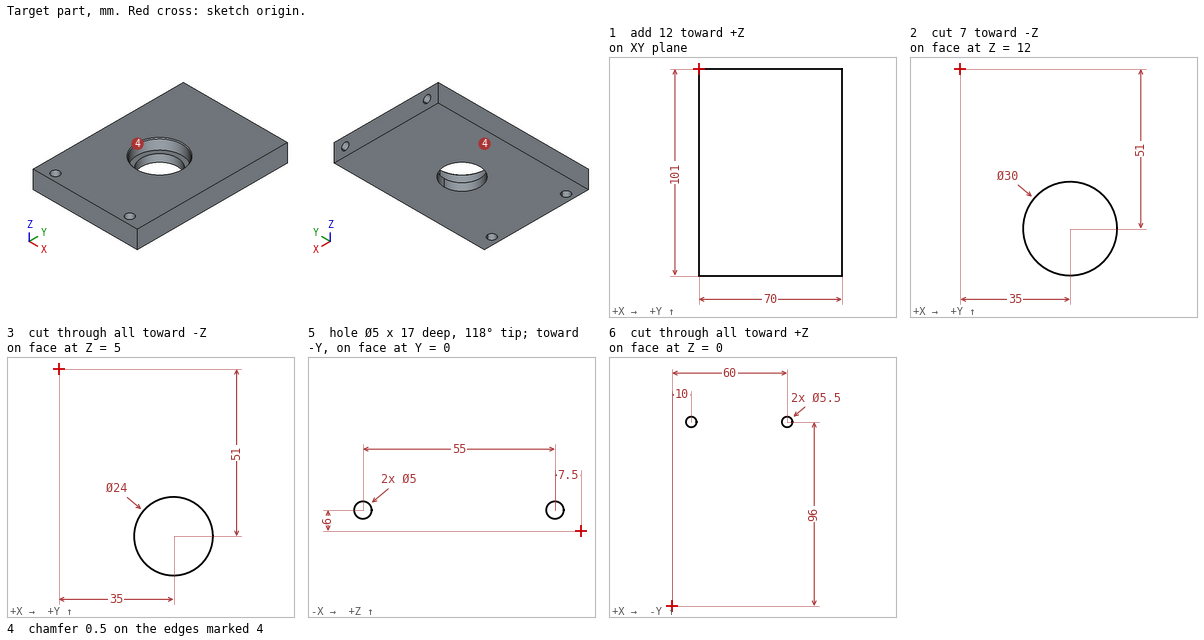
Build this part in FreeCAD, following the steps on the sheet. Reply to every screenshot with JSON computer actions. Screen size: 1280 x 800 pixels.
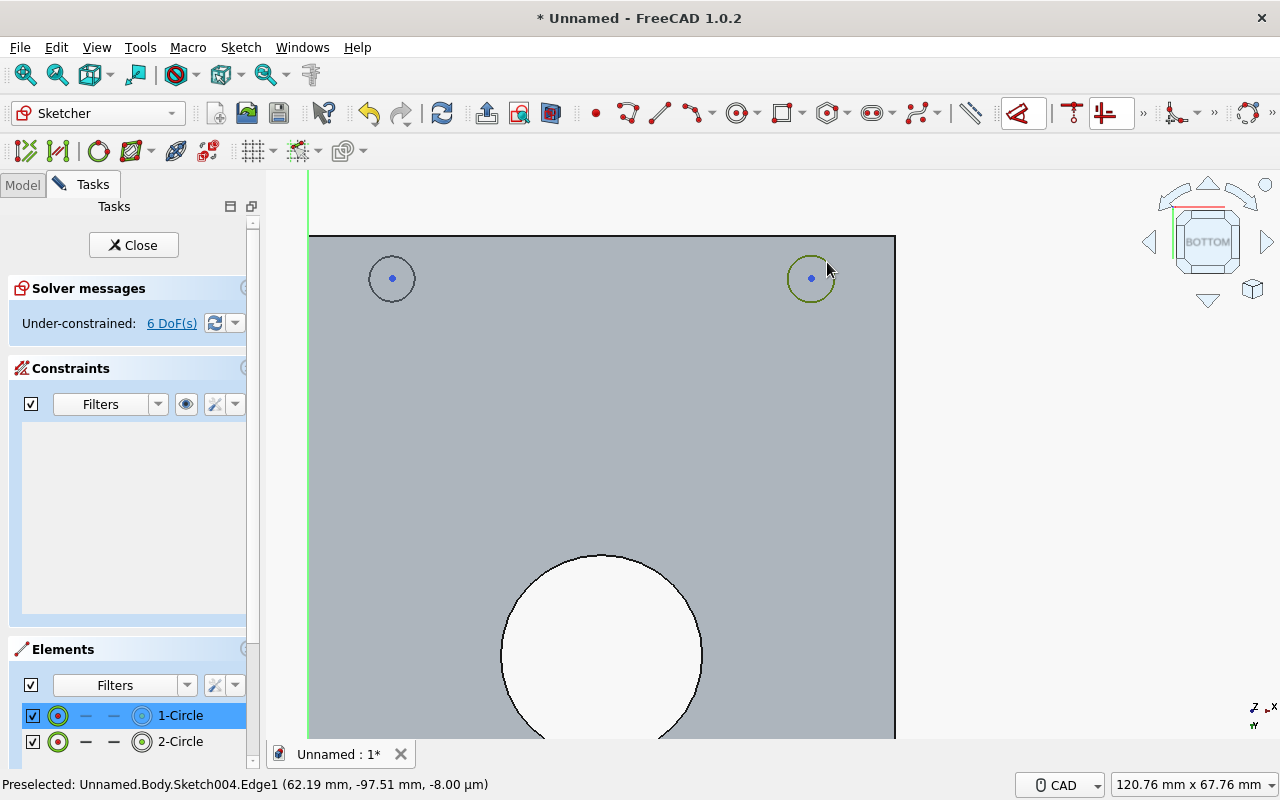
{"action": "left_click", "coordinate": [408, 263]}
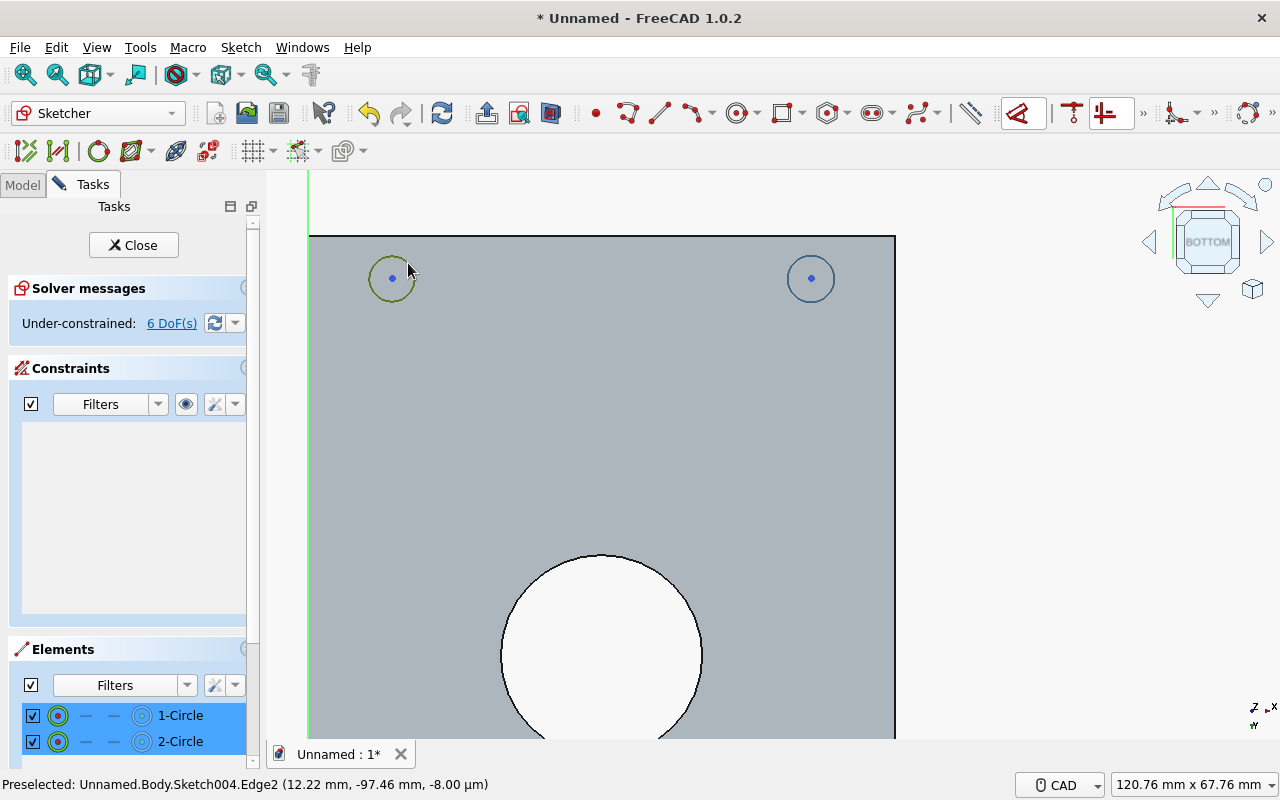
{"action": "key", "text": "e"}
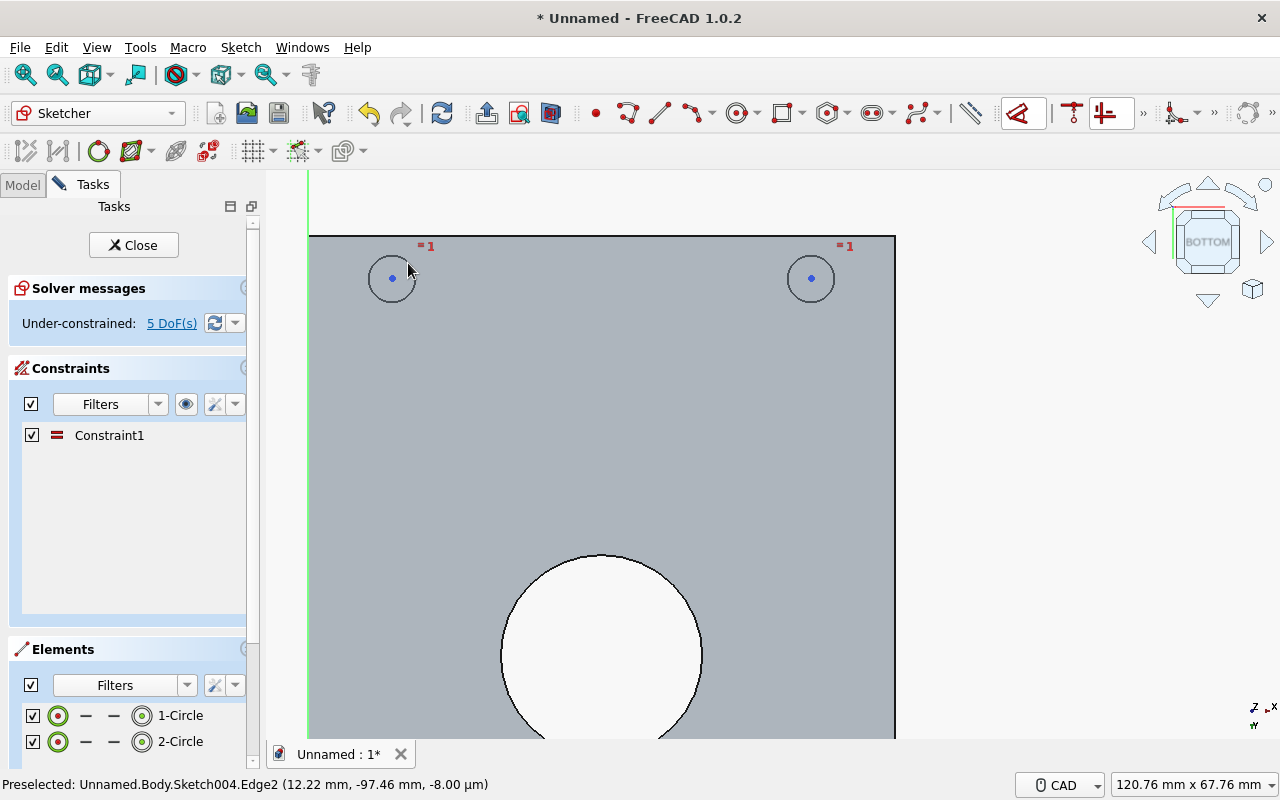
{"action": "left_click", "coordinate": [811, 279]}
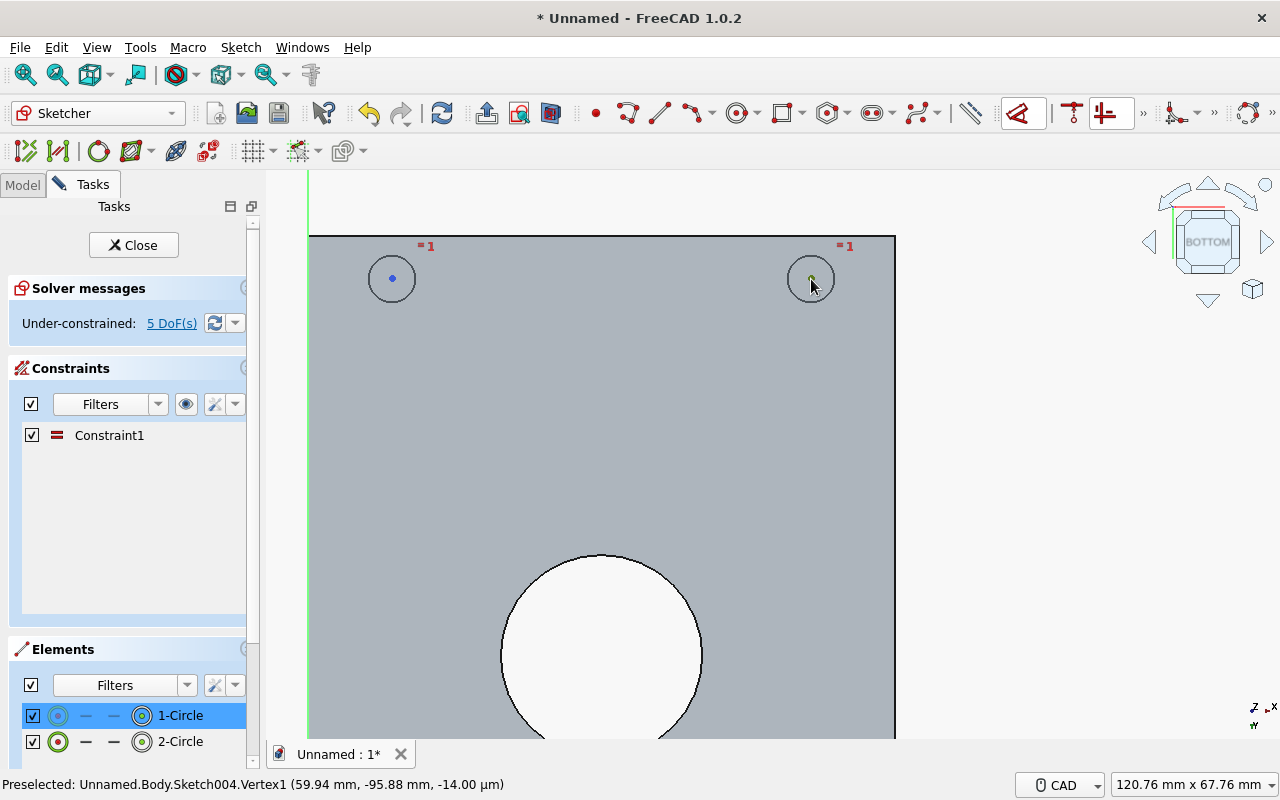
{"action": "left_click", "coordinate": [392, 279]}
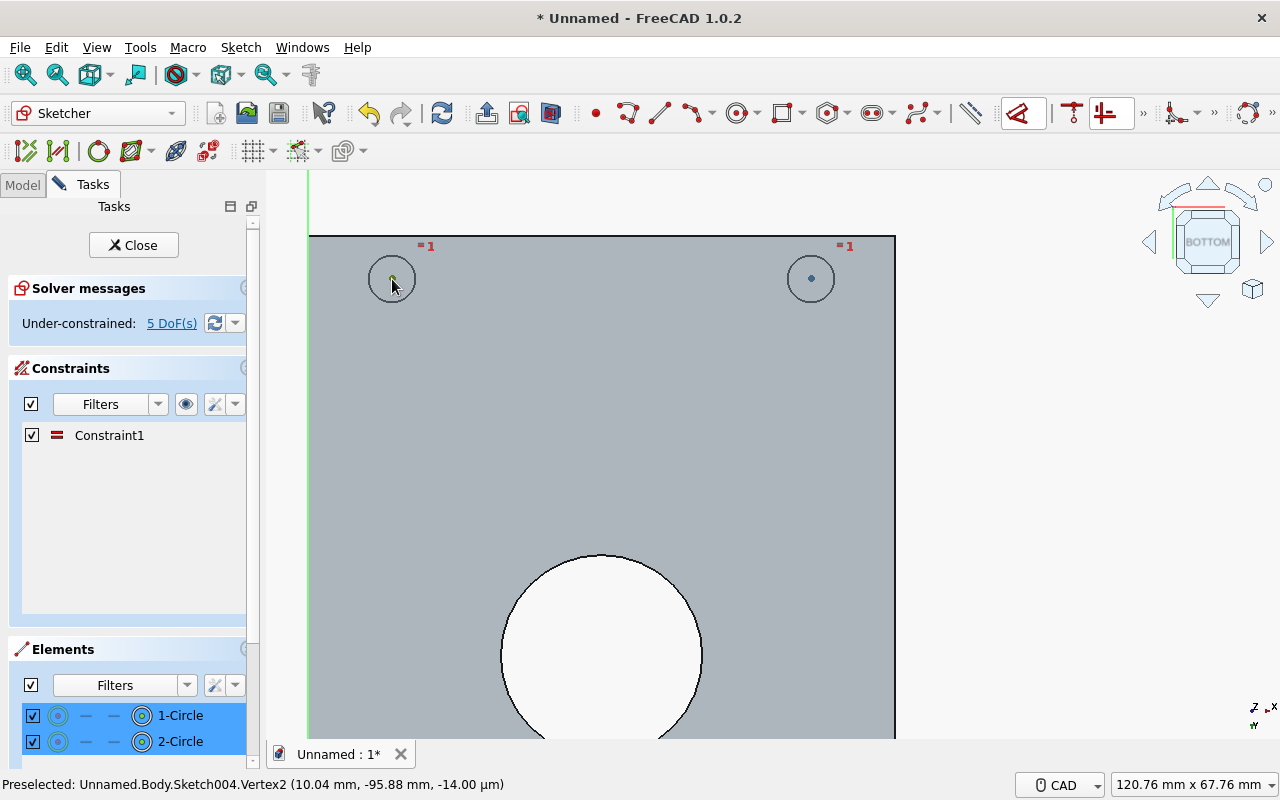
{"action": "key", "text": "h"}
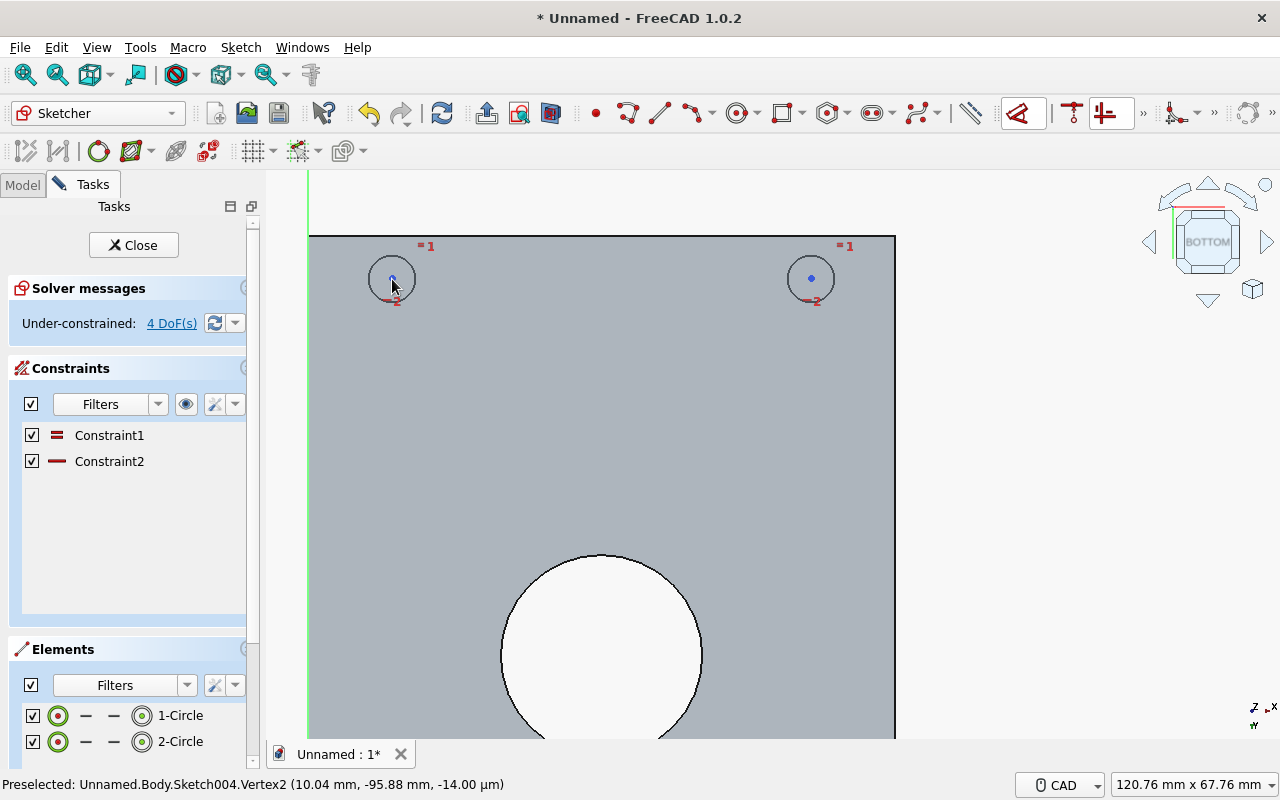
{"action": "left_click", "coordinate": [827, 262]}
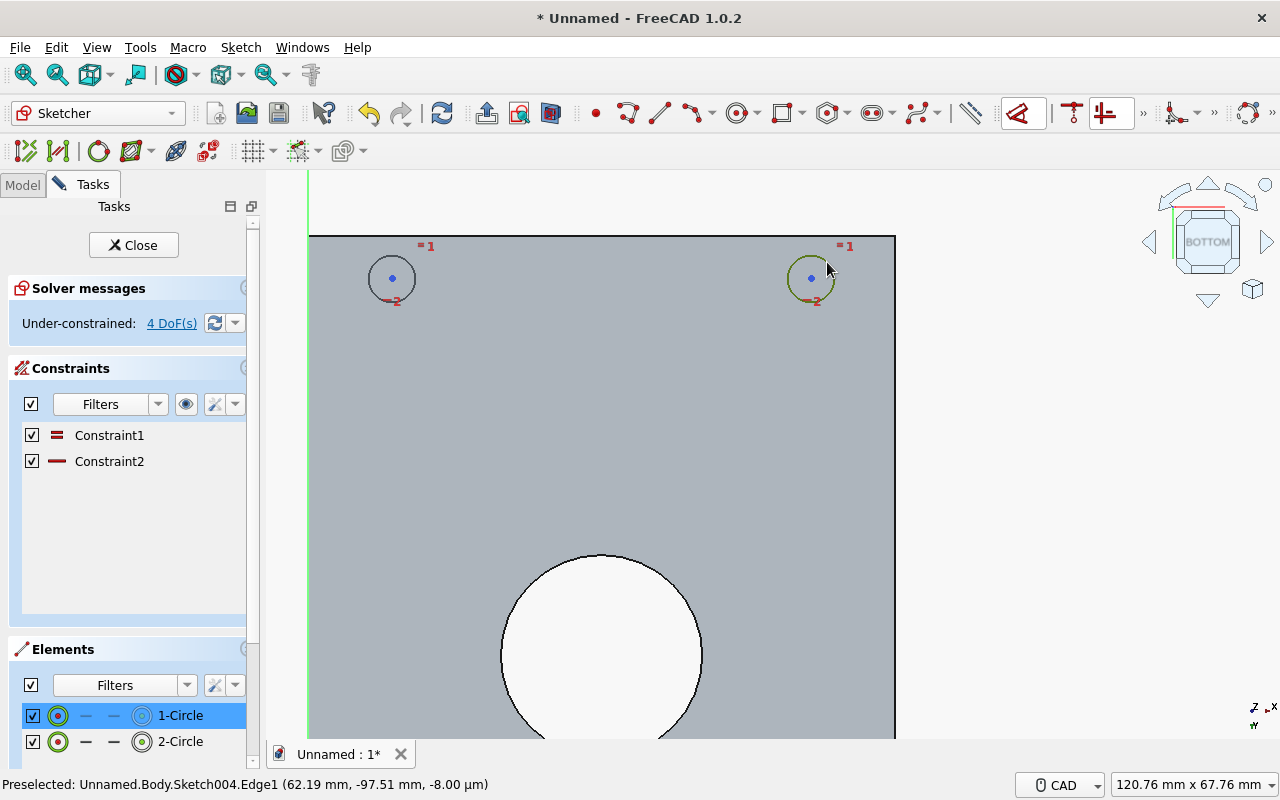
{"action": "key", "text": "k o"}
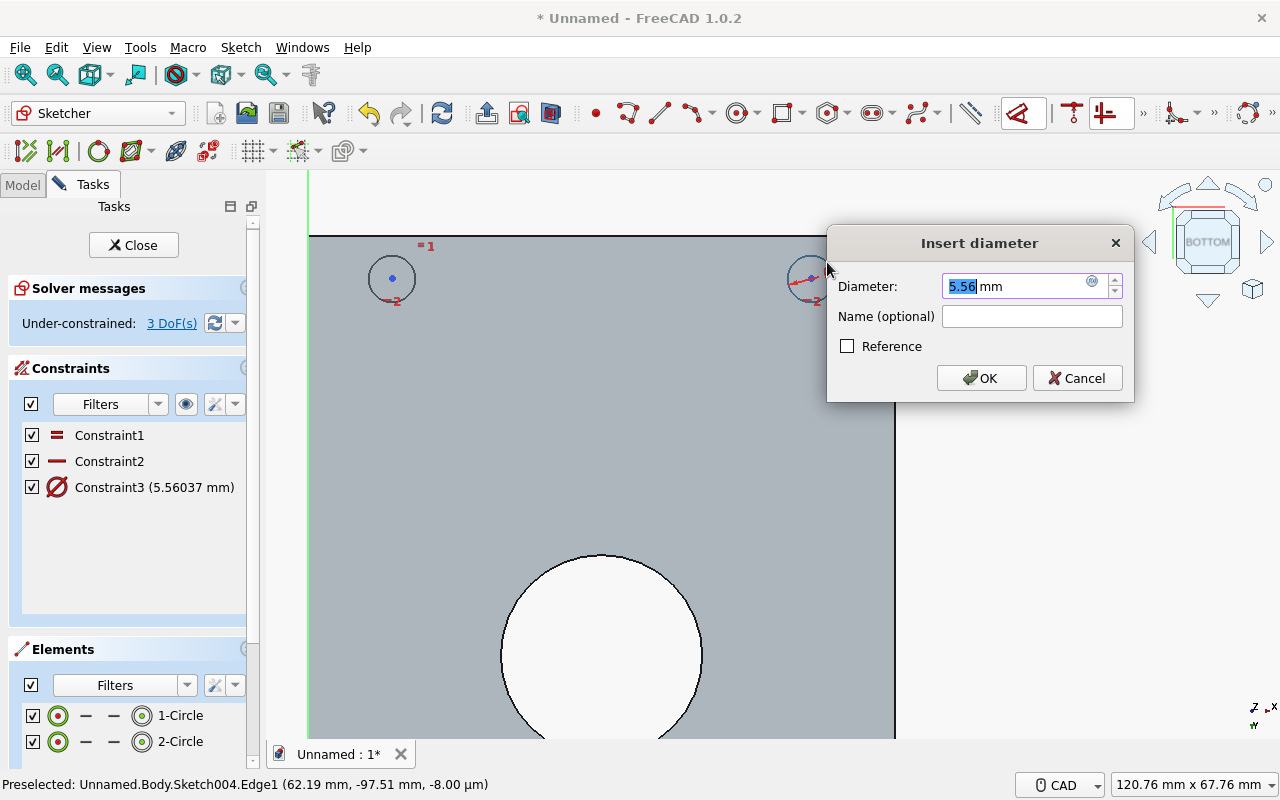
{"action": "type", "text": "5.5"}
{"action": "key", "text": "Return"}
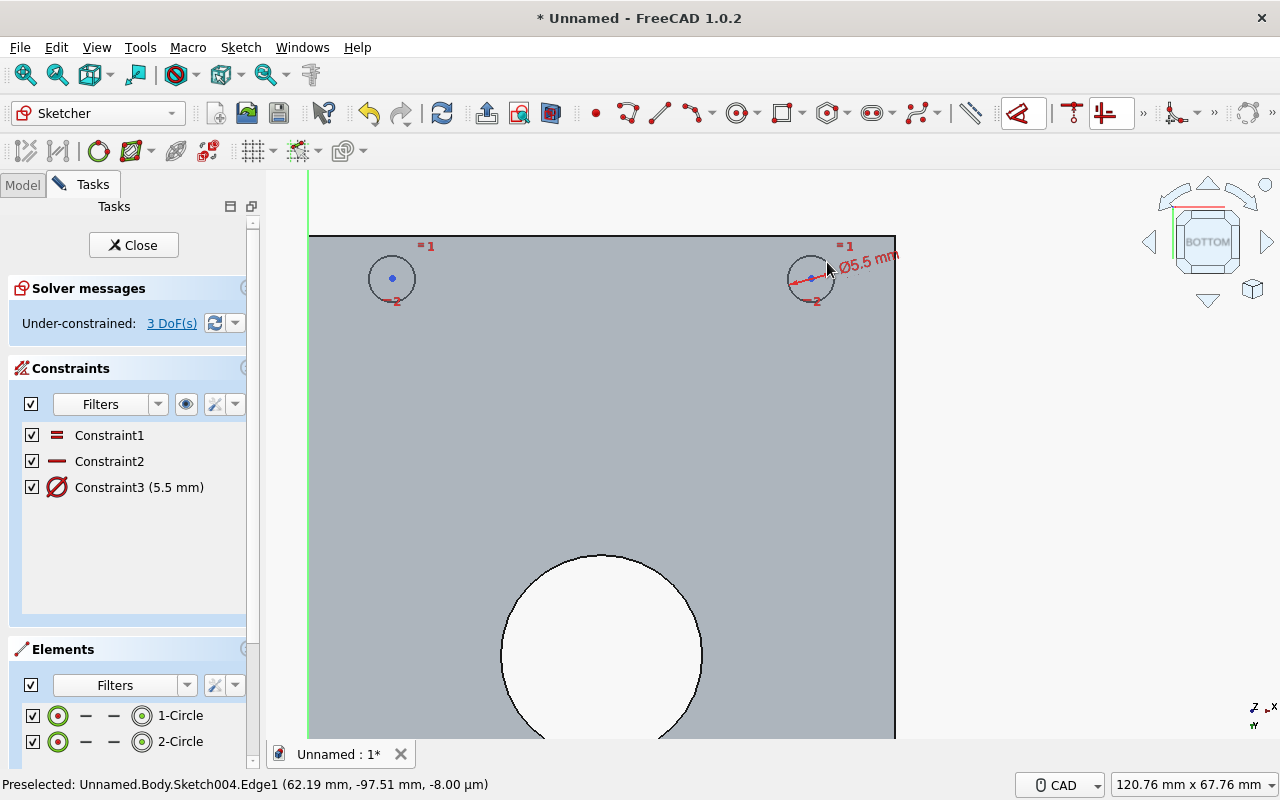
{"action": "left_click", "coordinate": [811, 279]}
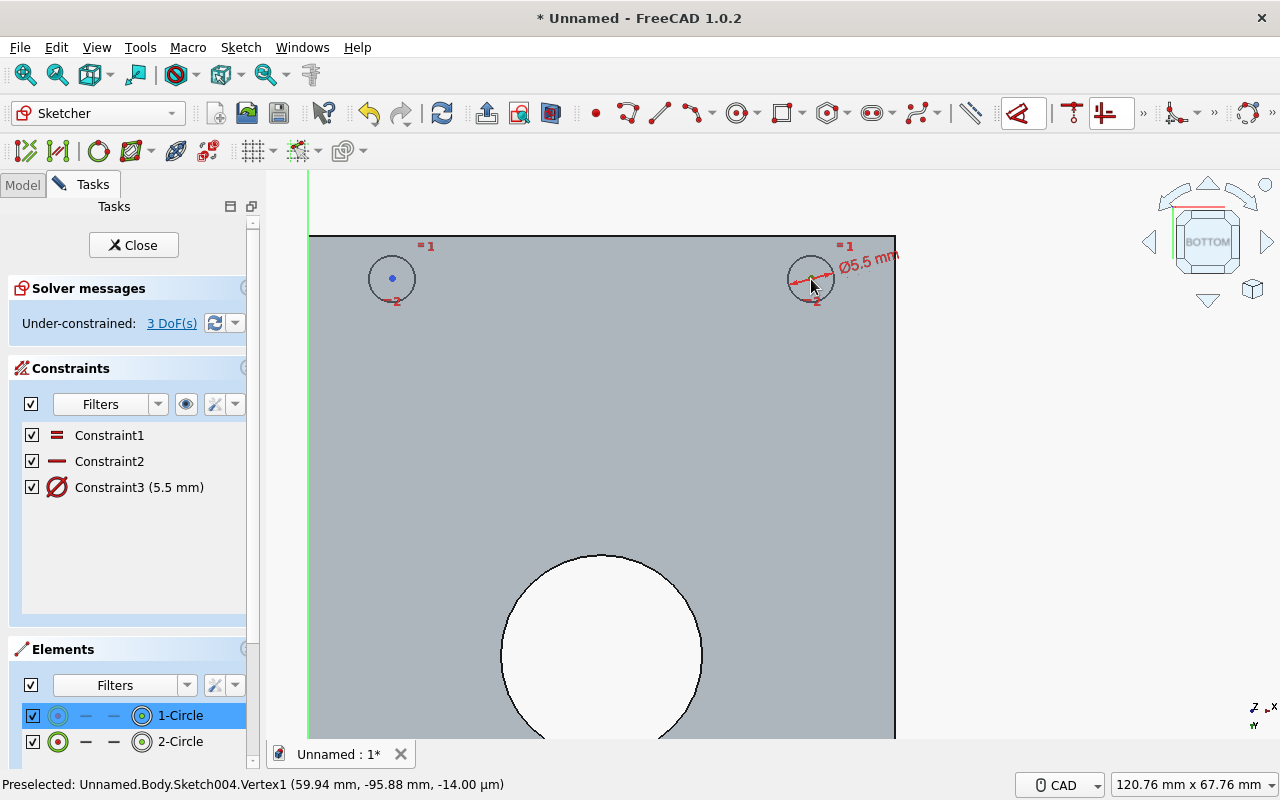
{"action": "key", "text": "l"}